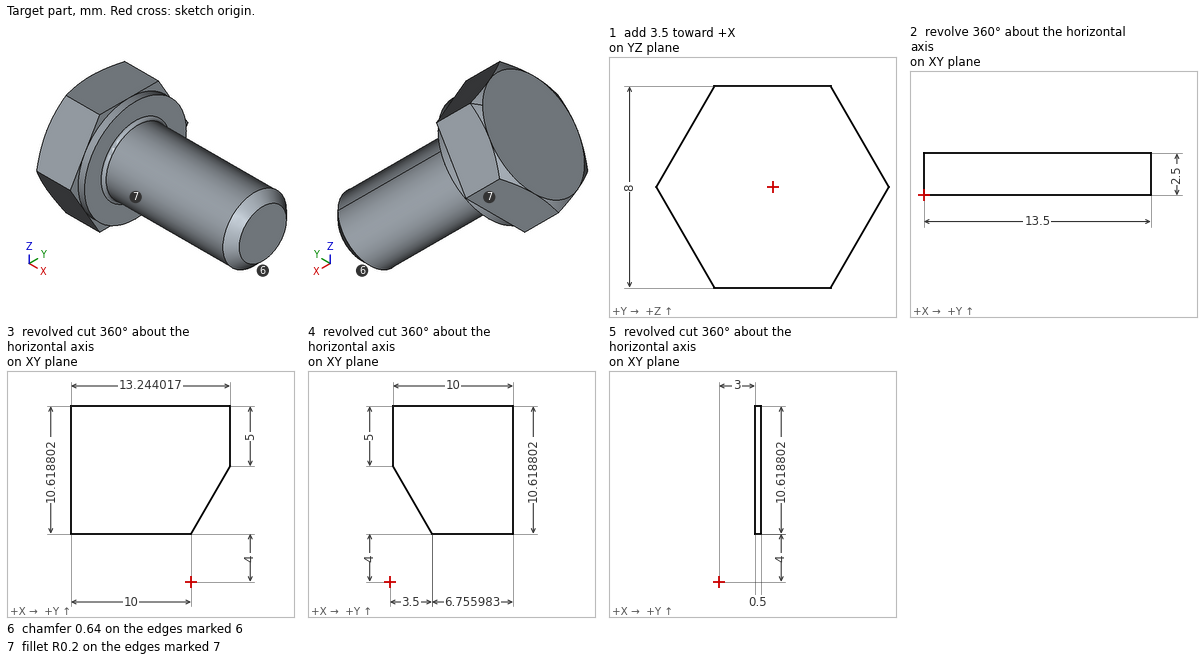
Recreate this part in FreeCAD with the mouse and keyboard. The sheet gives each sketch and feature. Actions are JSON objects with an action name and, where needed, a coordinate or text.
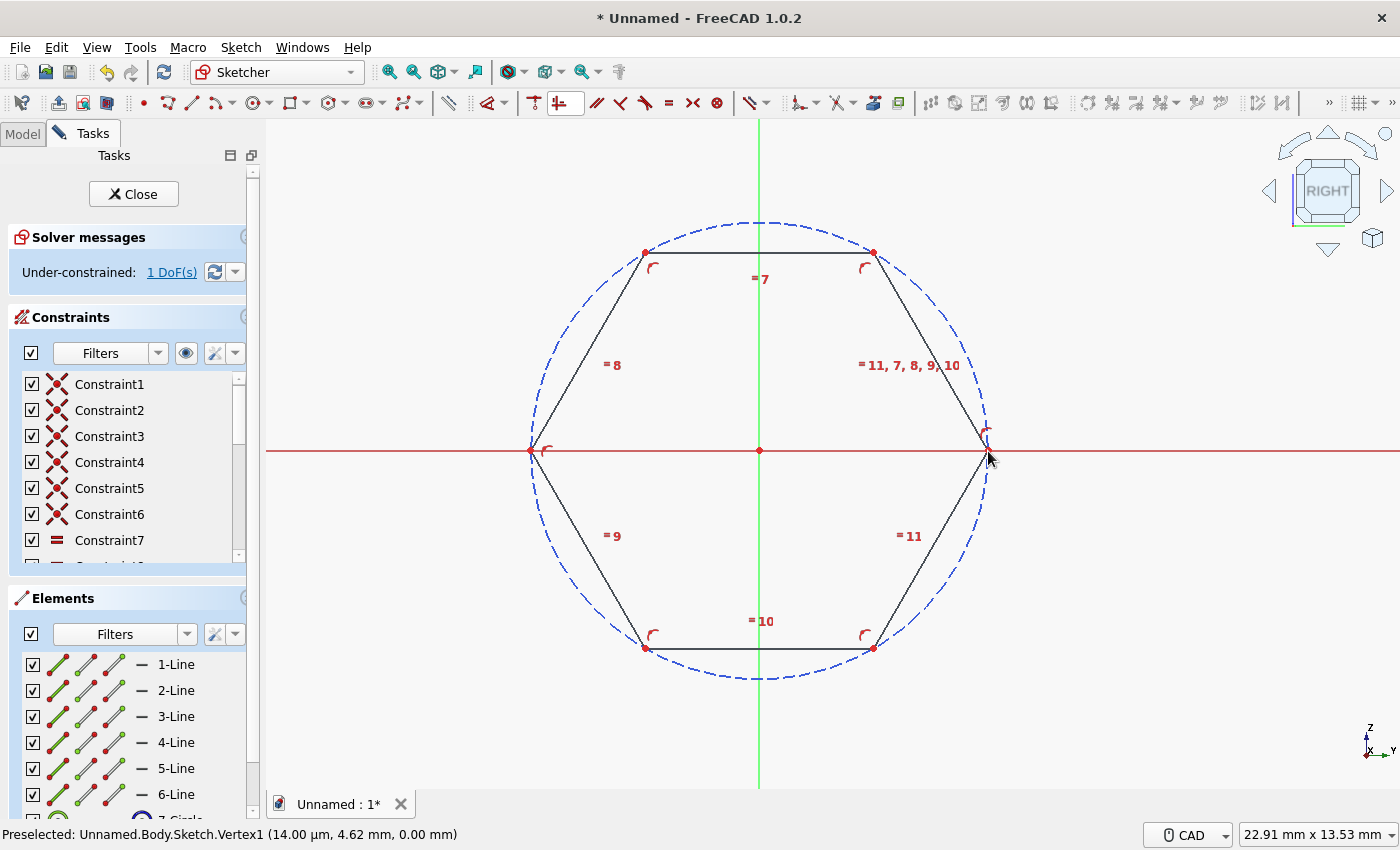
{"action": "left_click", "coordinate": [645, 649]}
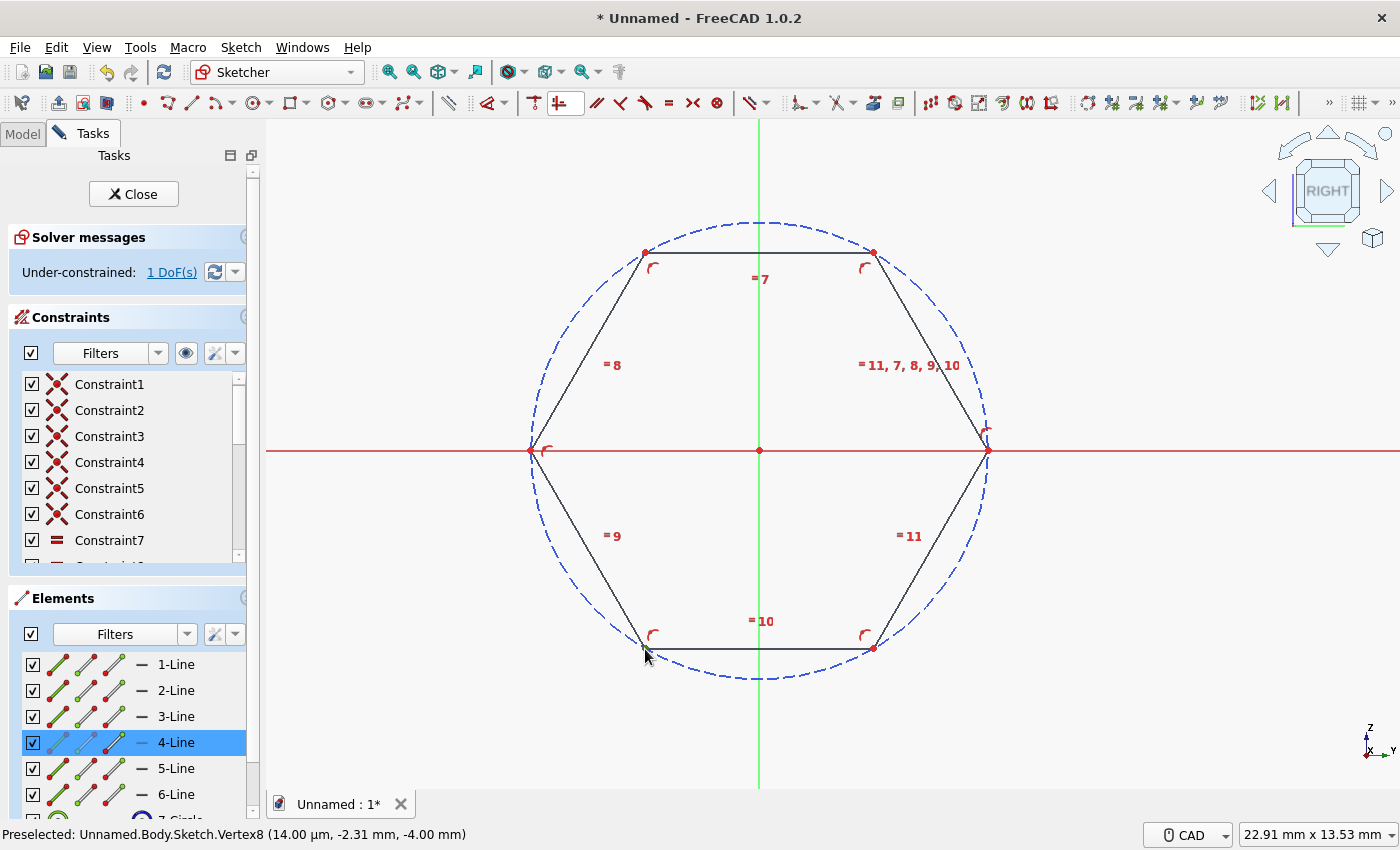
{"action": "left_click", "coordinate": [874, 253]}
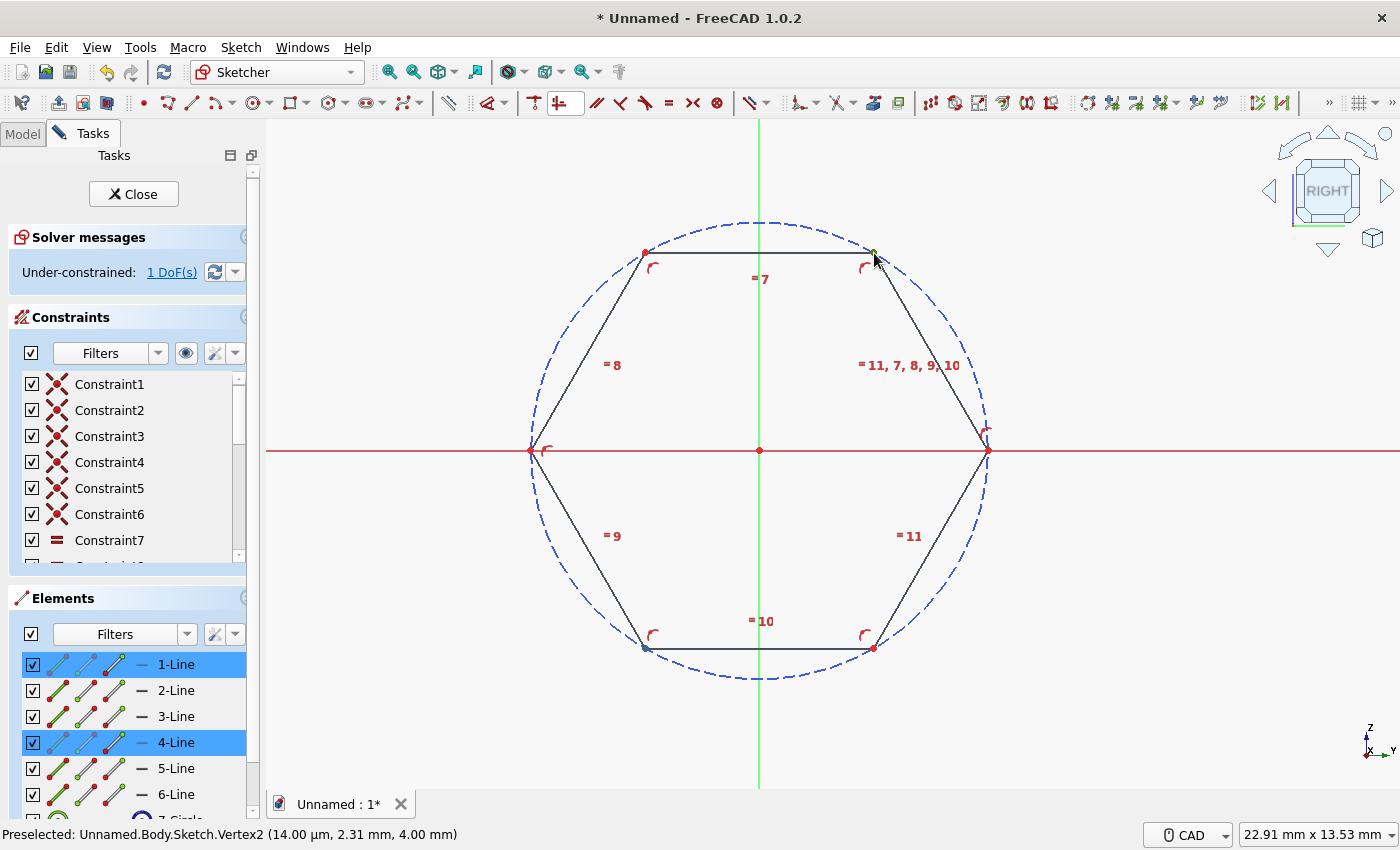
{"action": "key", "text": "i"}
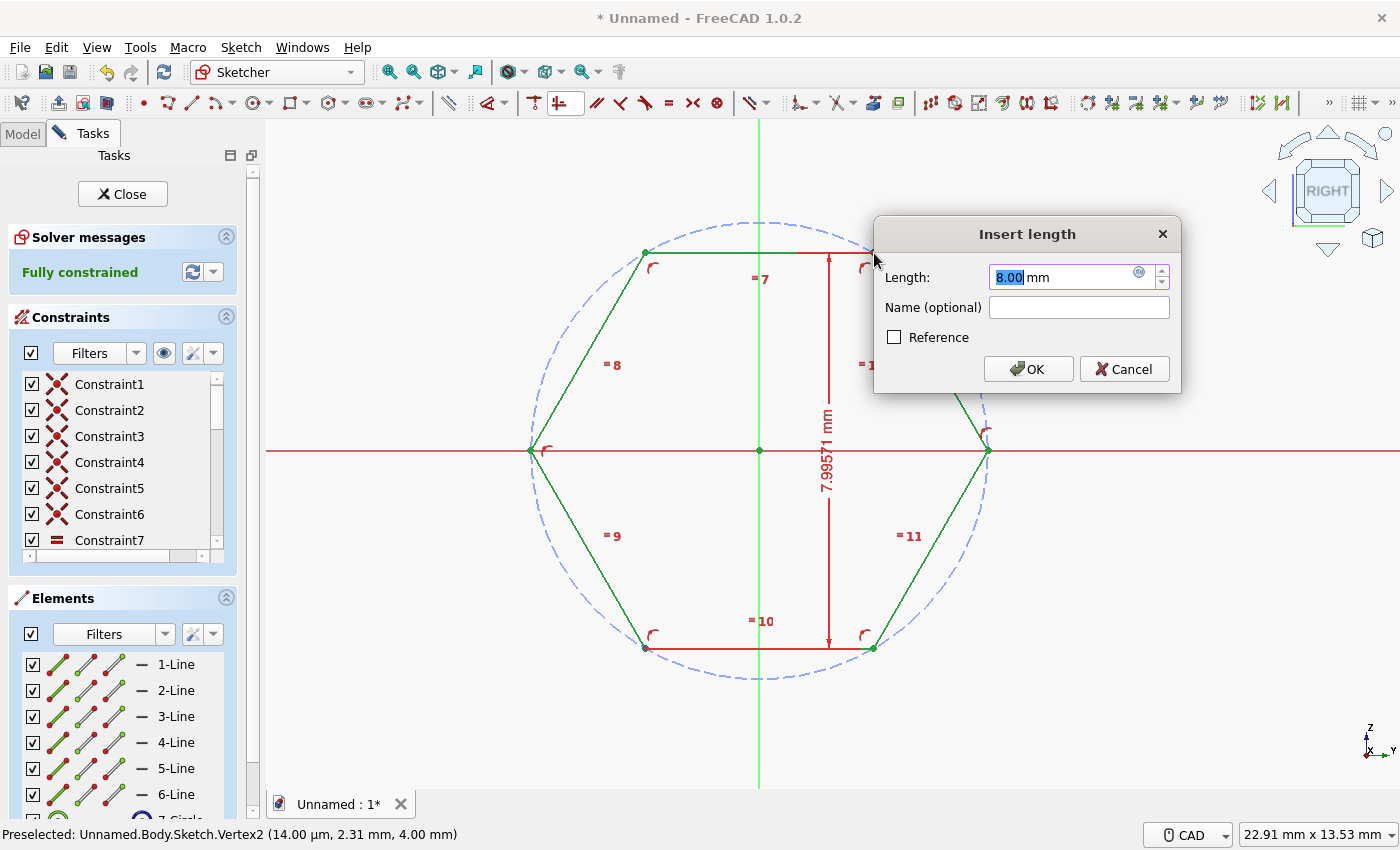
{"action": "type", "text": "8"}
{"action": "key", "text": "Return"}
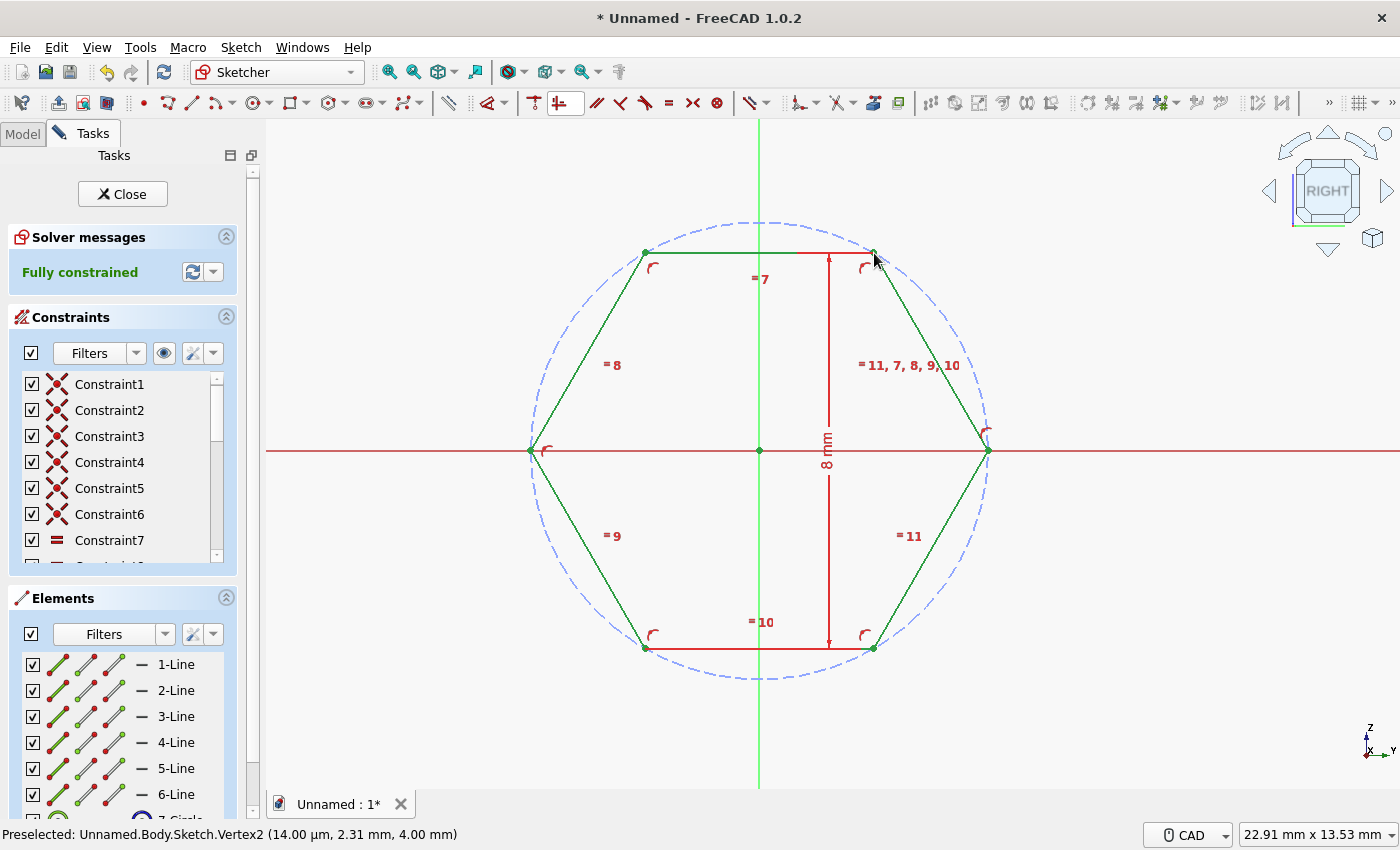
{"action": "left_click", "coordinate": [123, 194]}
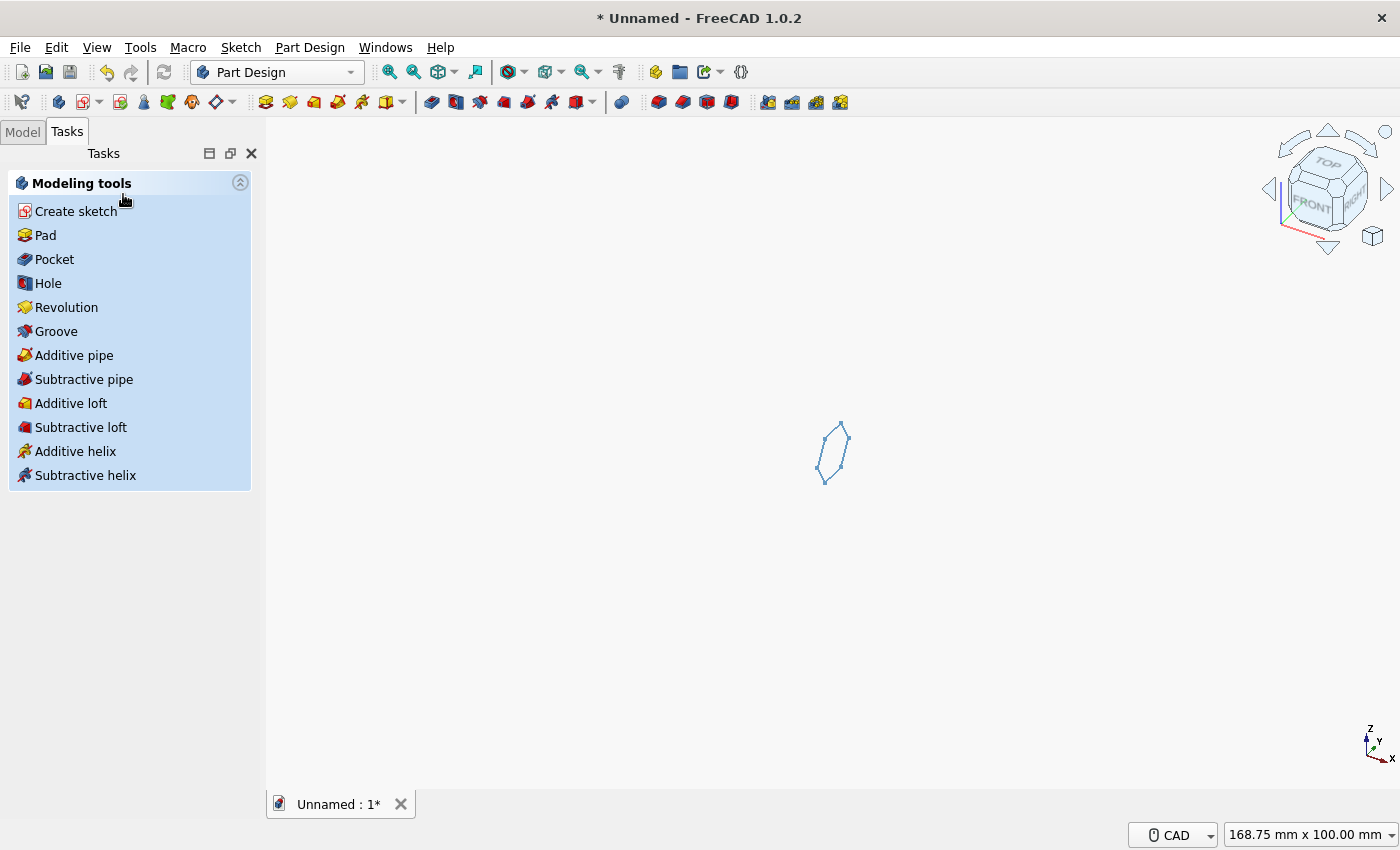
{"action": "left_click", "coordinate": [266, 102]}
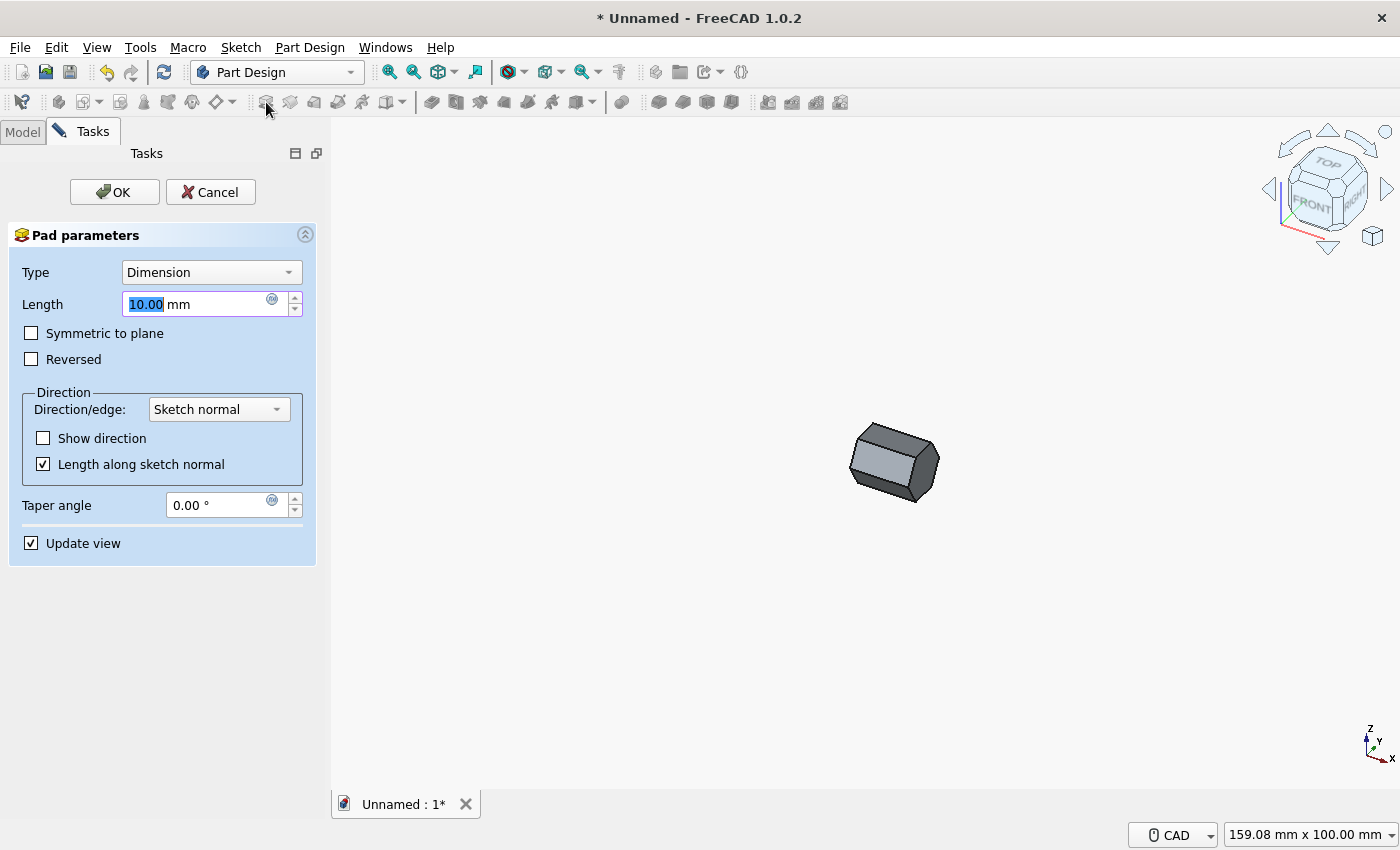
{"action": "type", "text": "3.5"}
{"action": "key", "text": "Tab"}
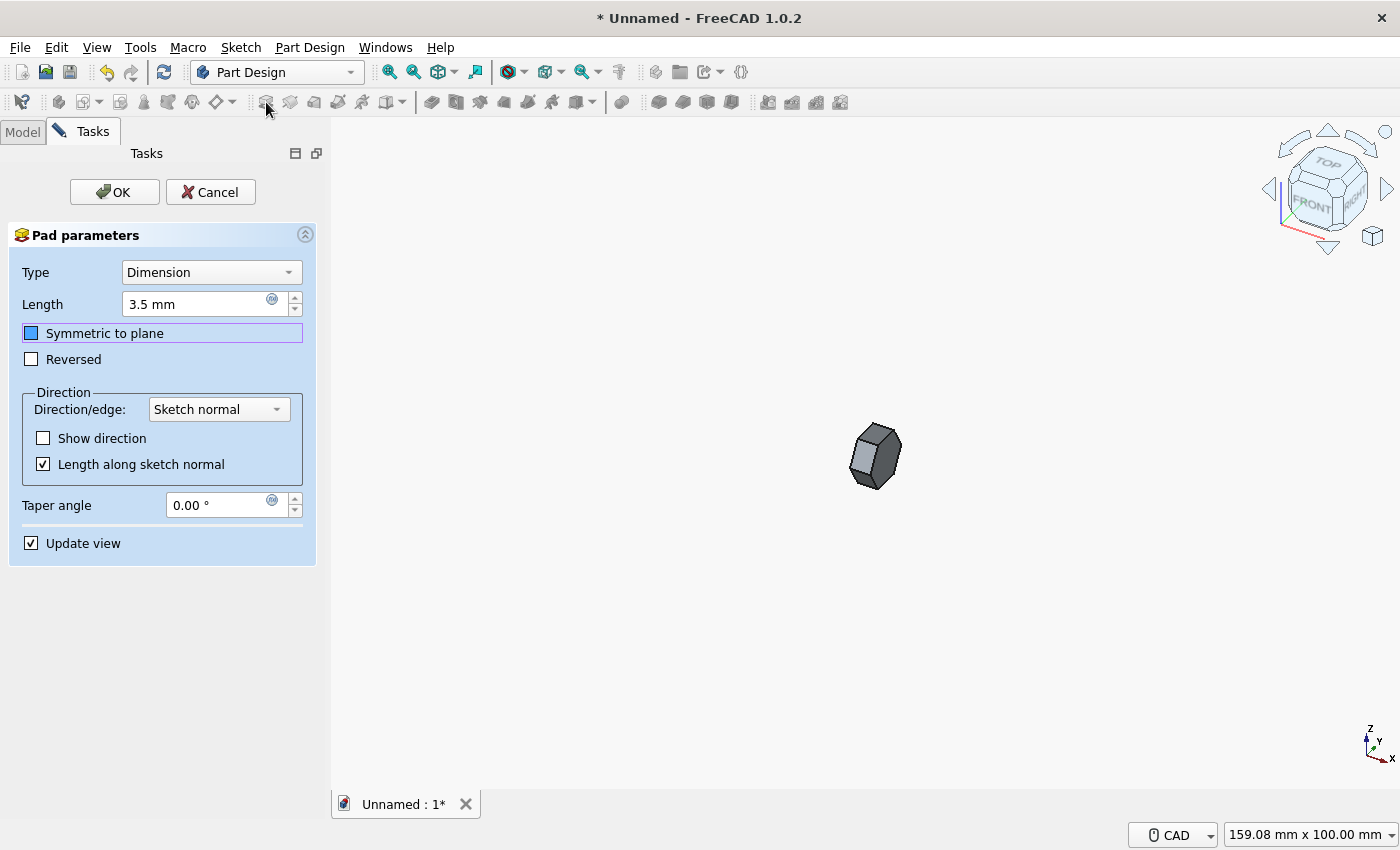
{"action": "left_click", "coordinate": [115, 192]}